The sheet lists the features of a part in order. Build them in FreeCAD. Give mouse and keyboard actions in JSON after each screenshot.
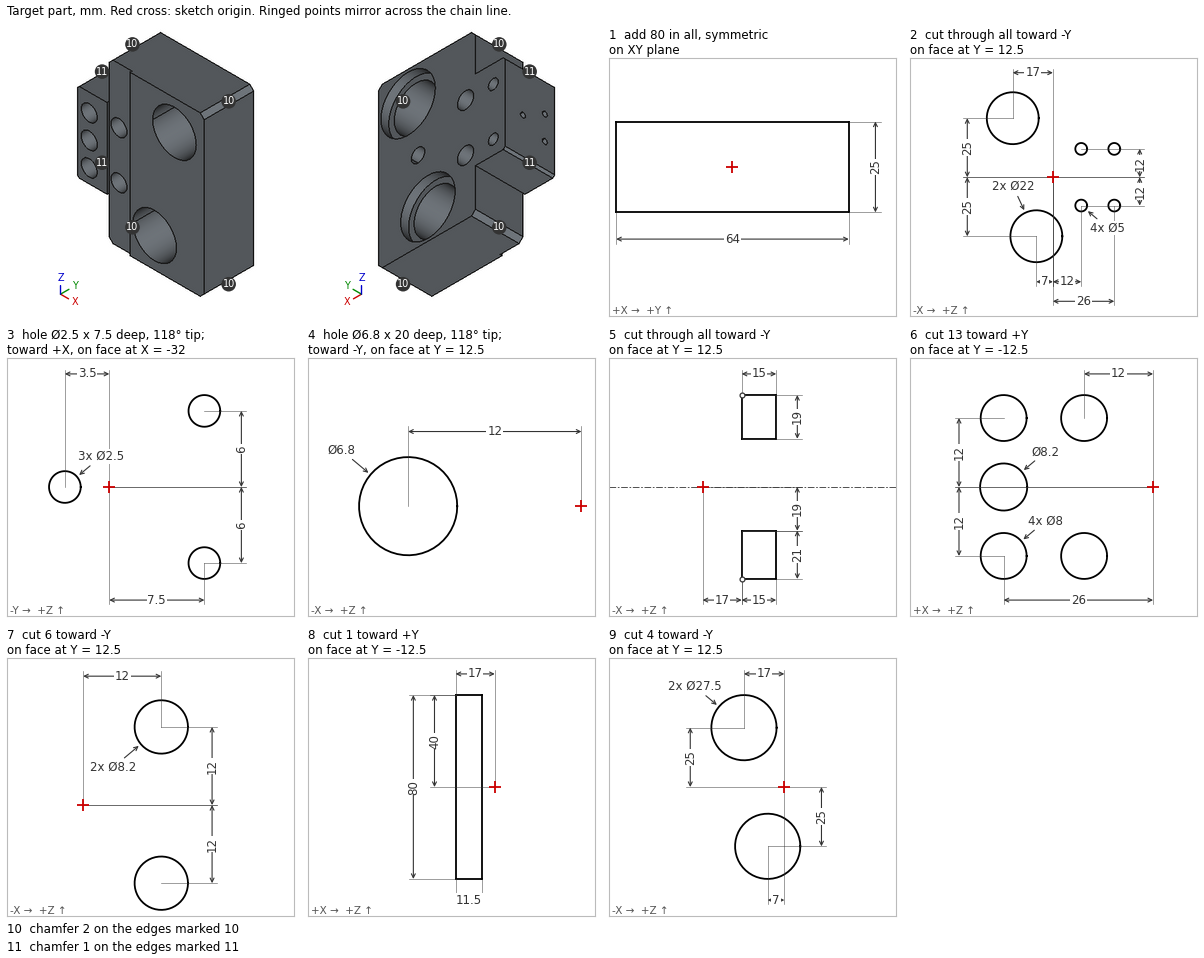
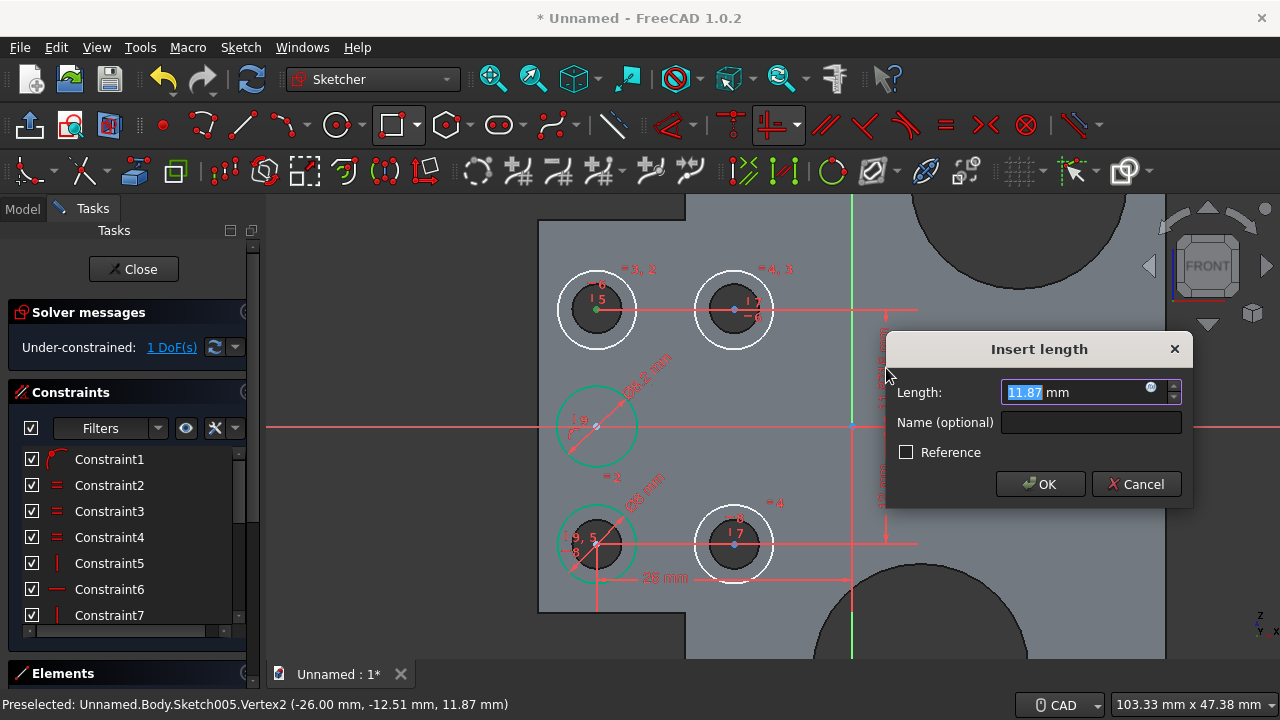
{"action": "type", "text": "12"}
{"action": "key", "text": "Return"}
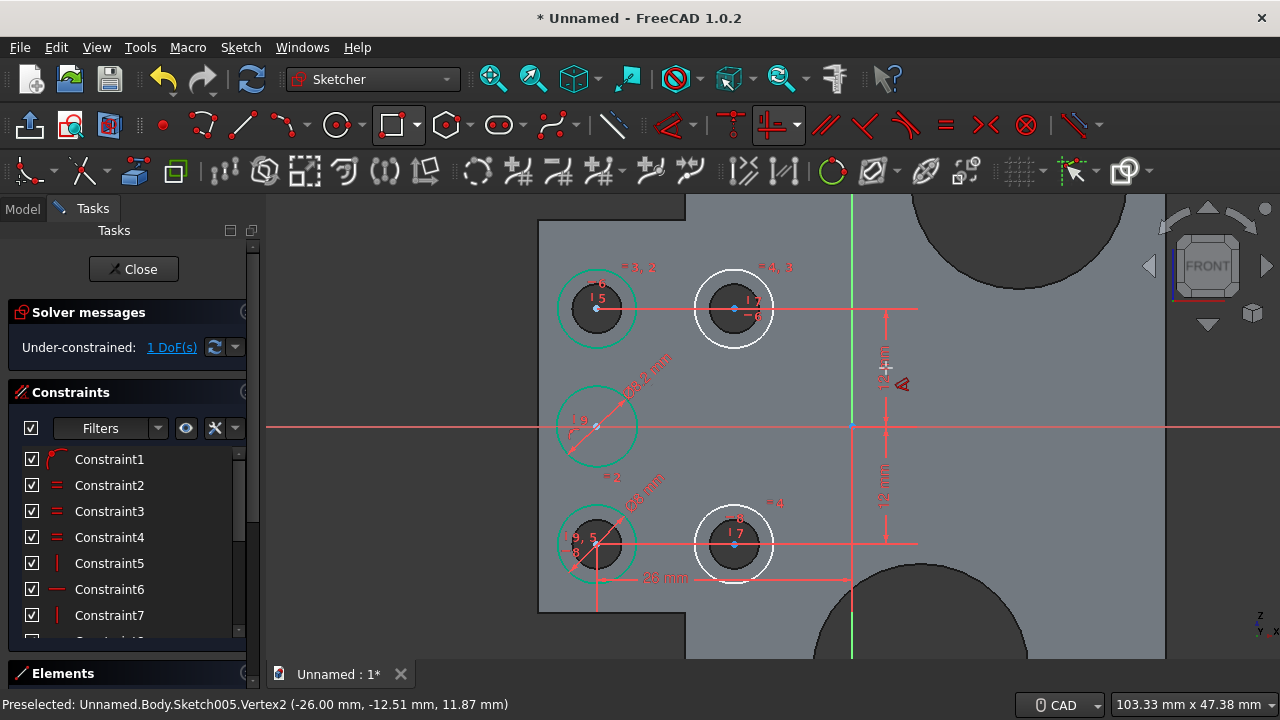
{"action": "left_click", "coordinate": [734, 309]}
{"action": "left_click", "coordinate": [793, 275]}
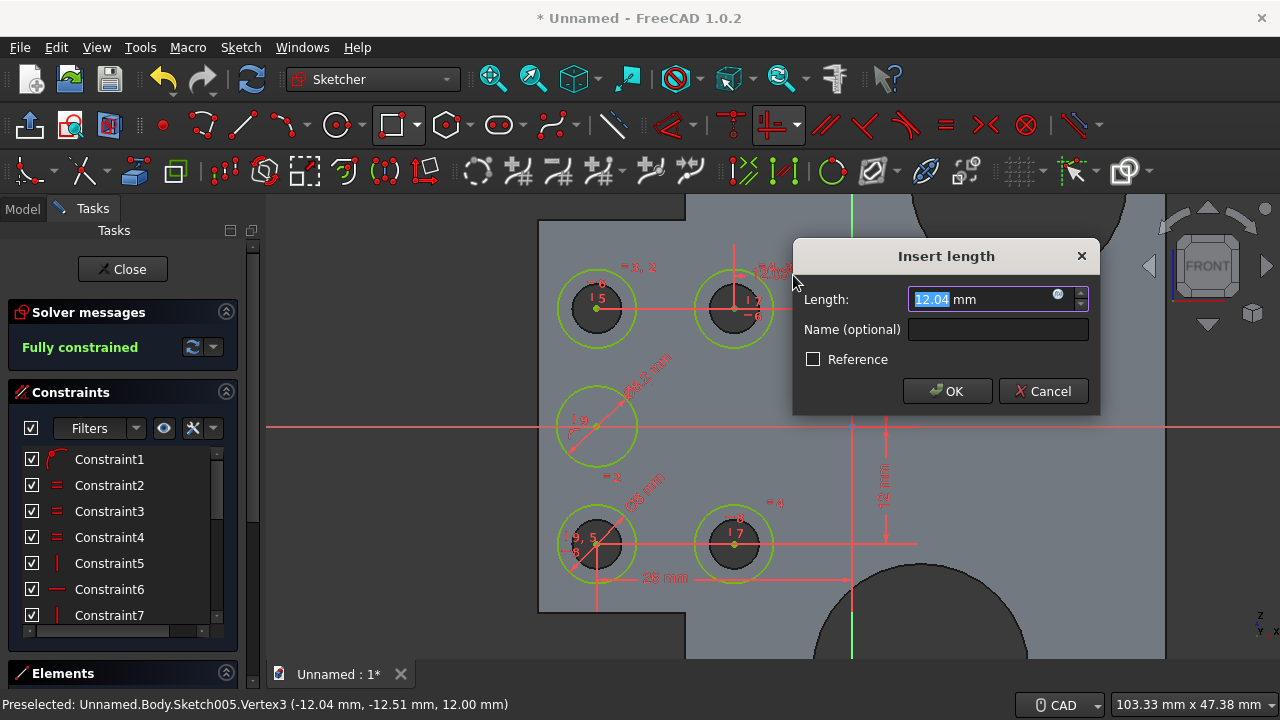
{"action": "type", "text": "12"}
{"action": "key", "text": "Return"}
{"action": "key", "text": "Escape"}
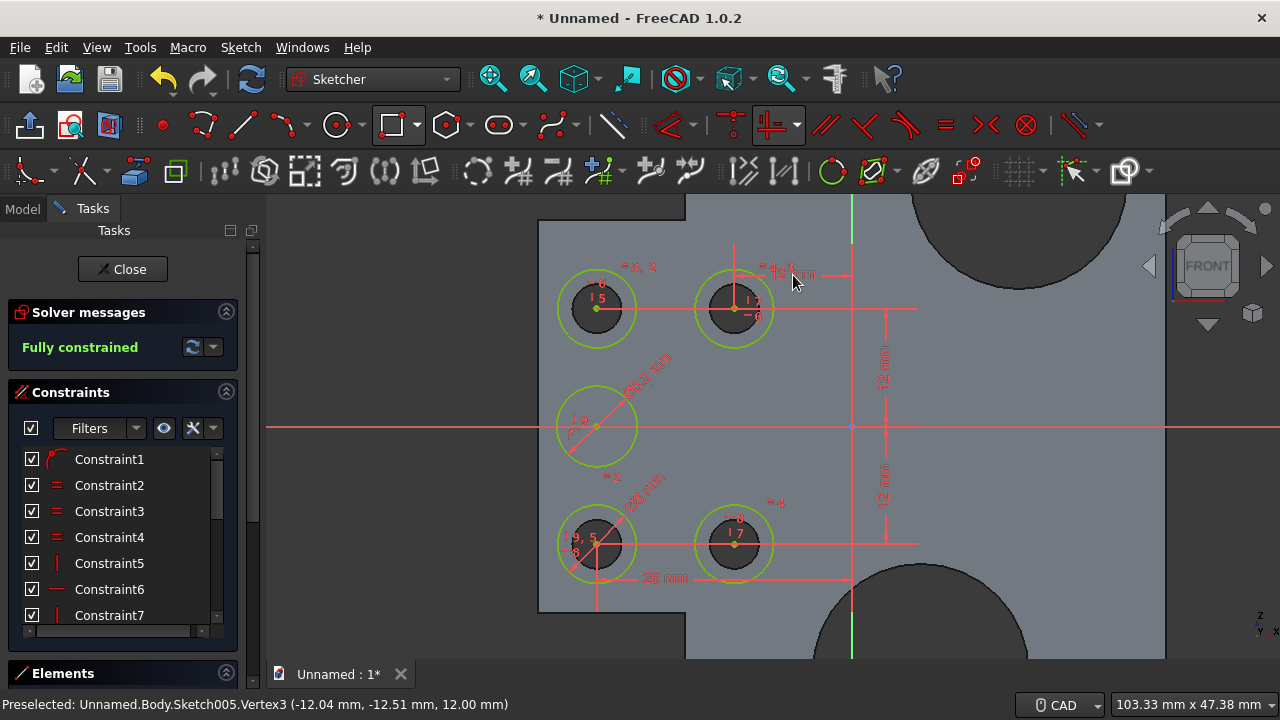
{"action": "left_click", "coordinate": [123, 269]}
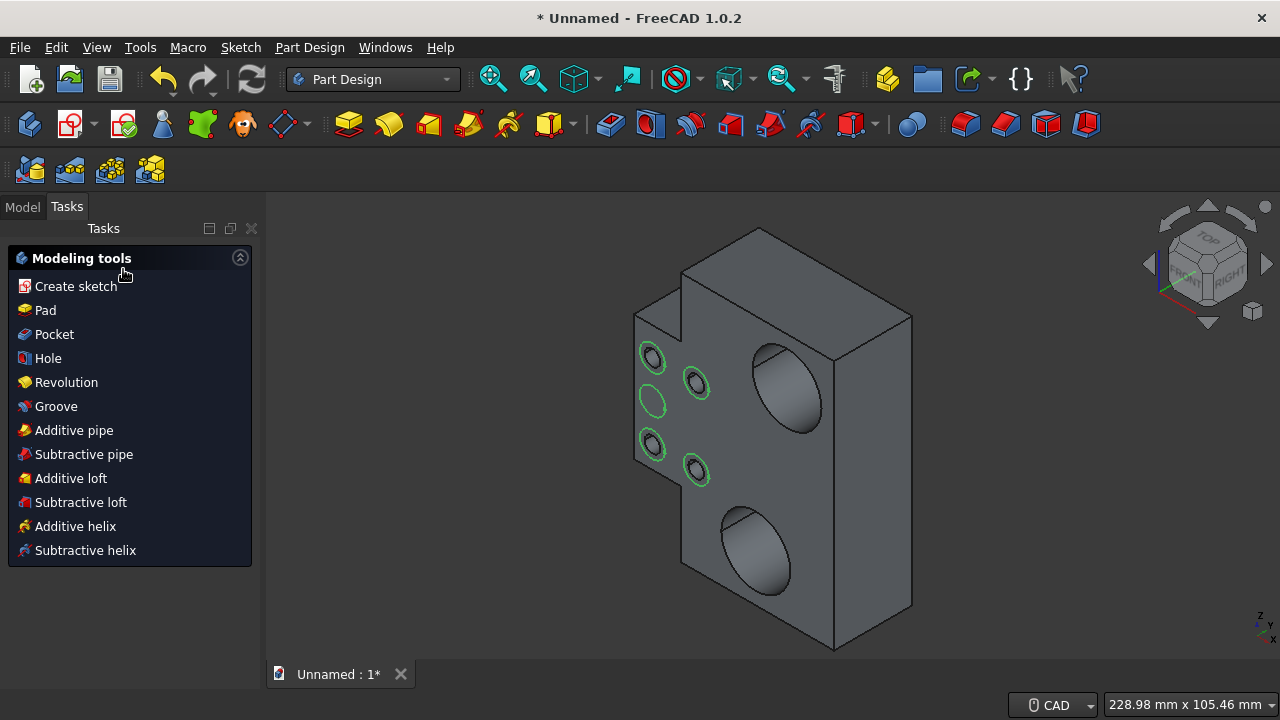
{"action": "left_click", "coordinate": [612, 124]}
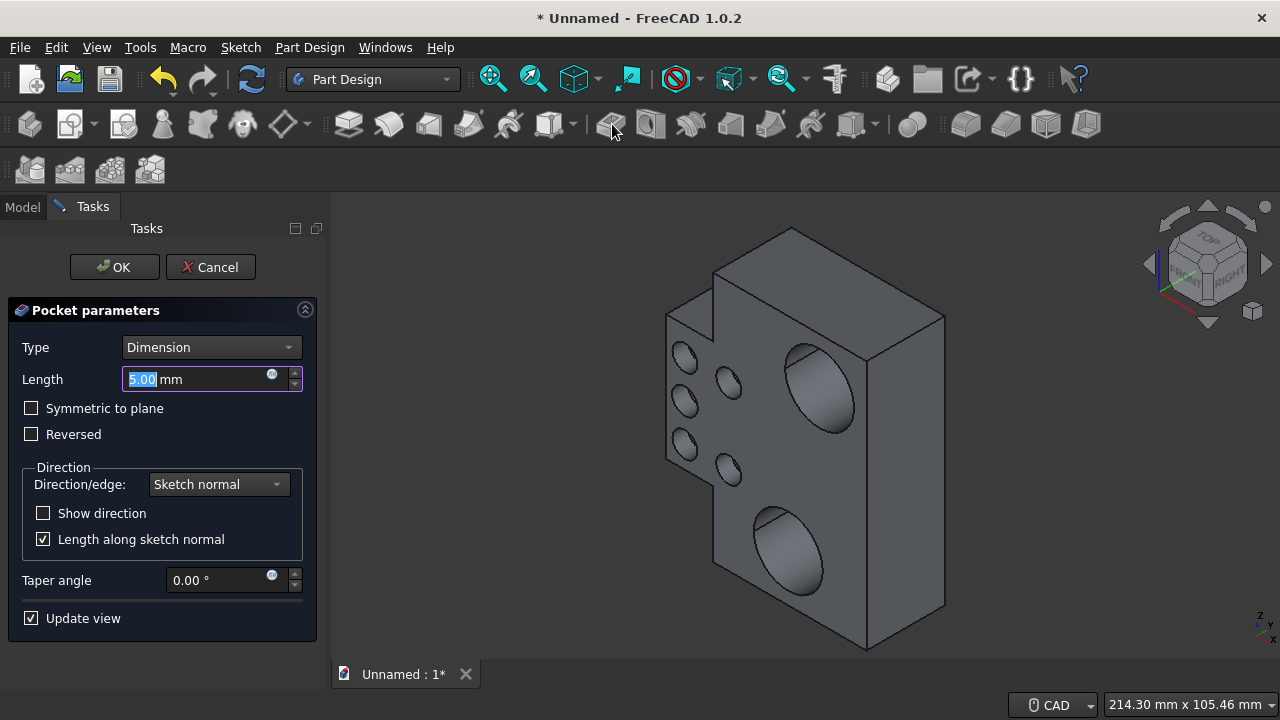
{"action": "type", "text": "13"}
{"action": "key", "text": "Tab"}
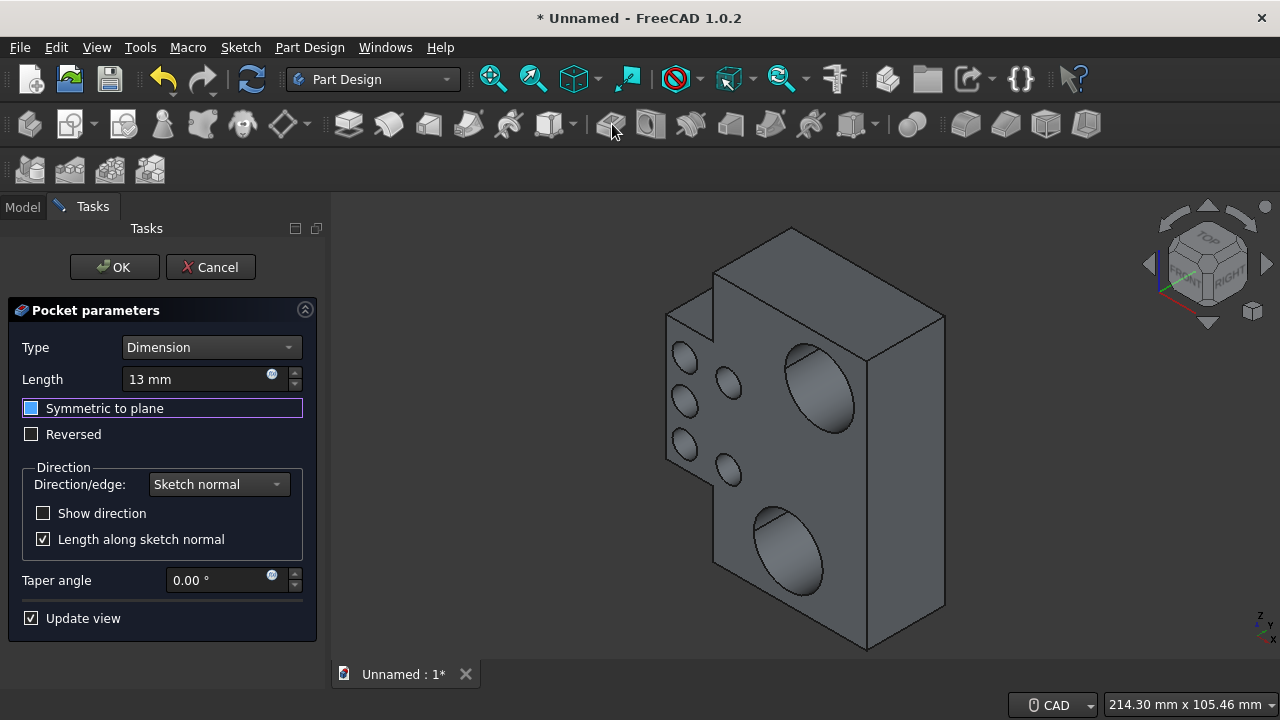
{"action": "left_click", "coordinate": [115, 267]}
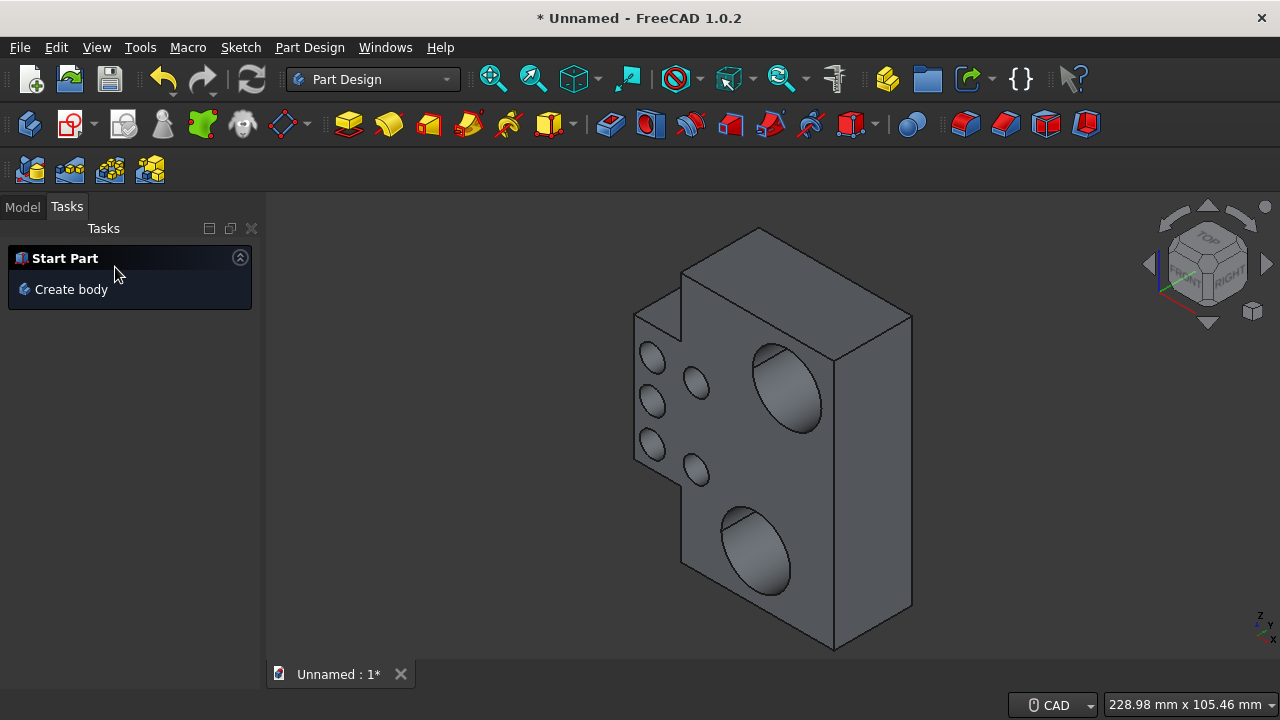
{"action": "key", "text": "4"}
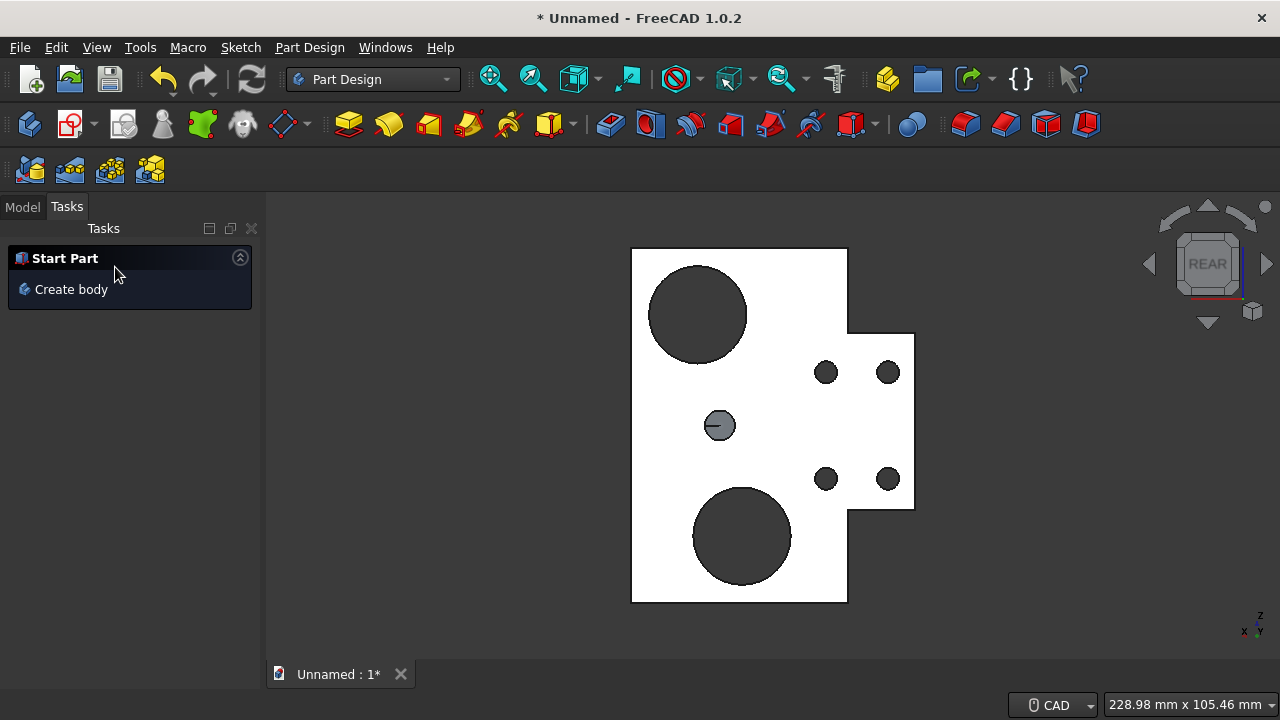
{"action": "left_click", "coordinate": [854, 424]}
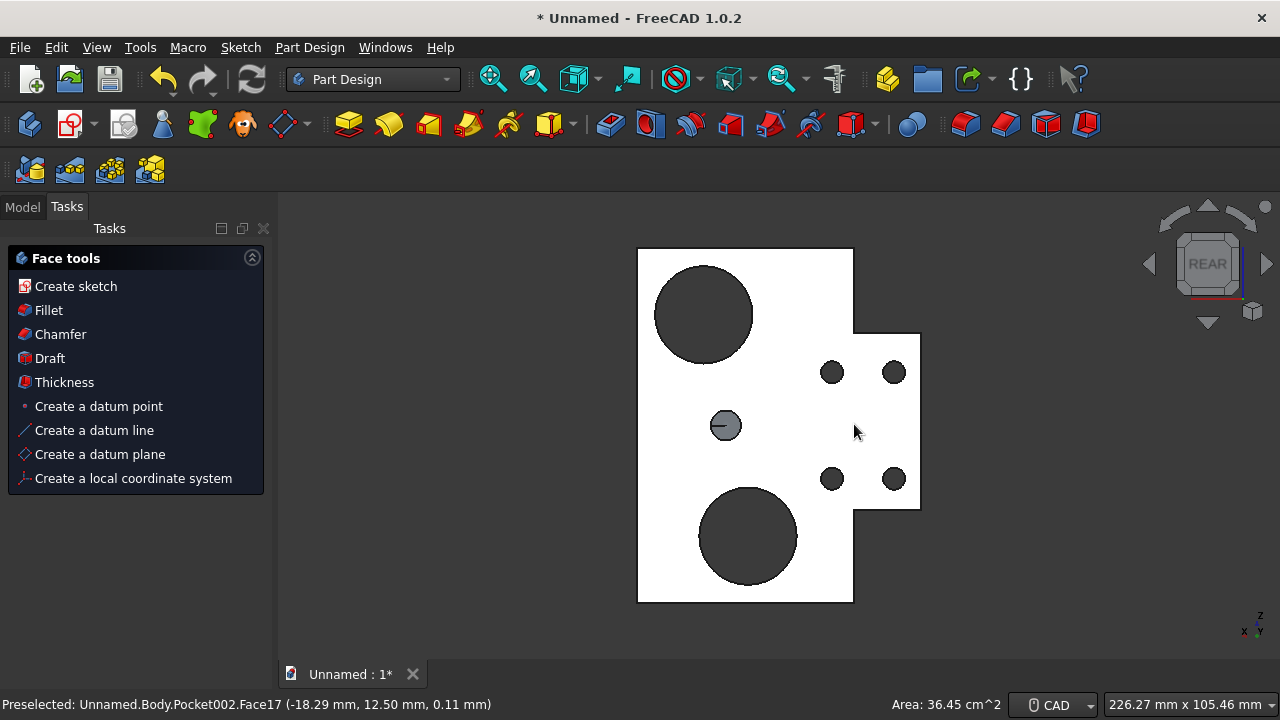
{"action": "left_click", "coordinate": [70, 124]}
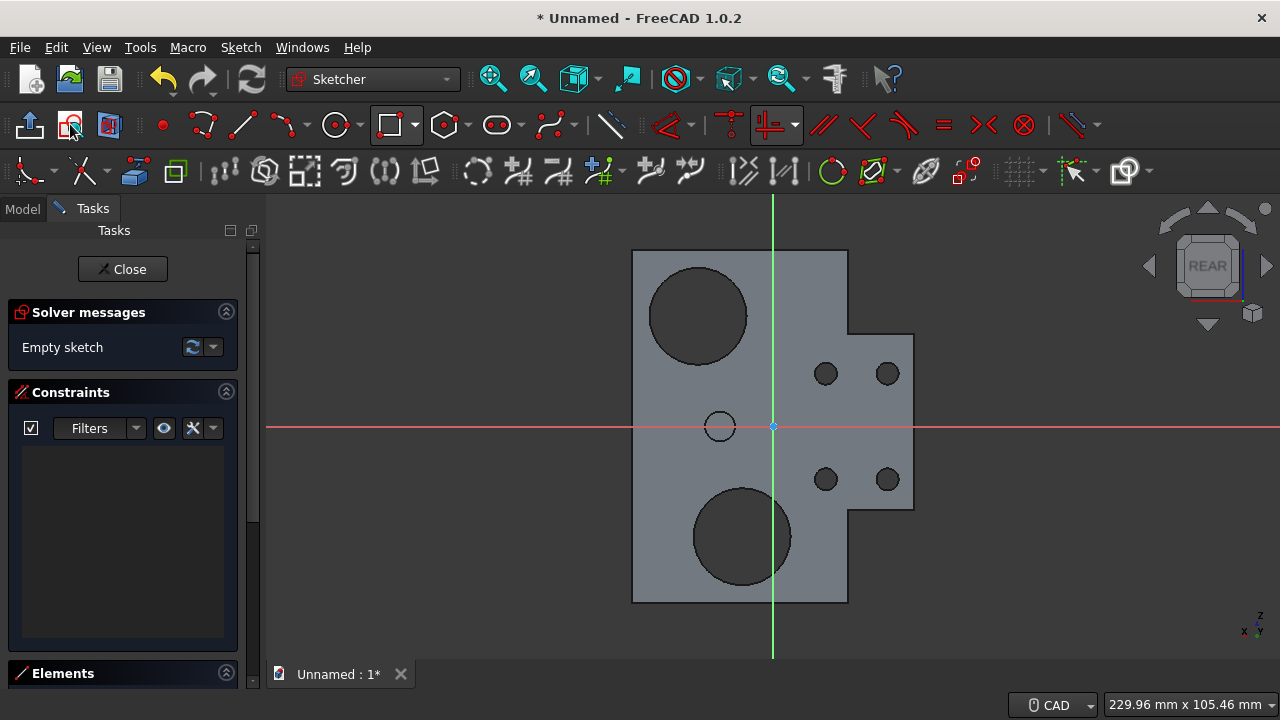
{"action": "scroll", "coordinate": [893, 426], "scroll_direction": "up", "scroll_amount": 4}